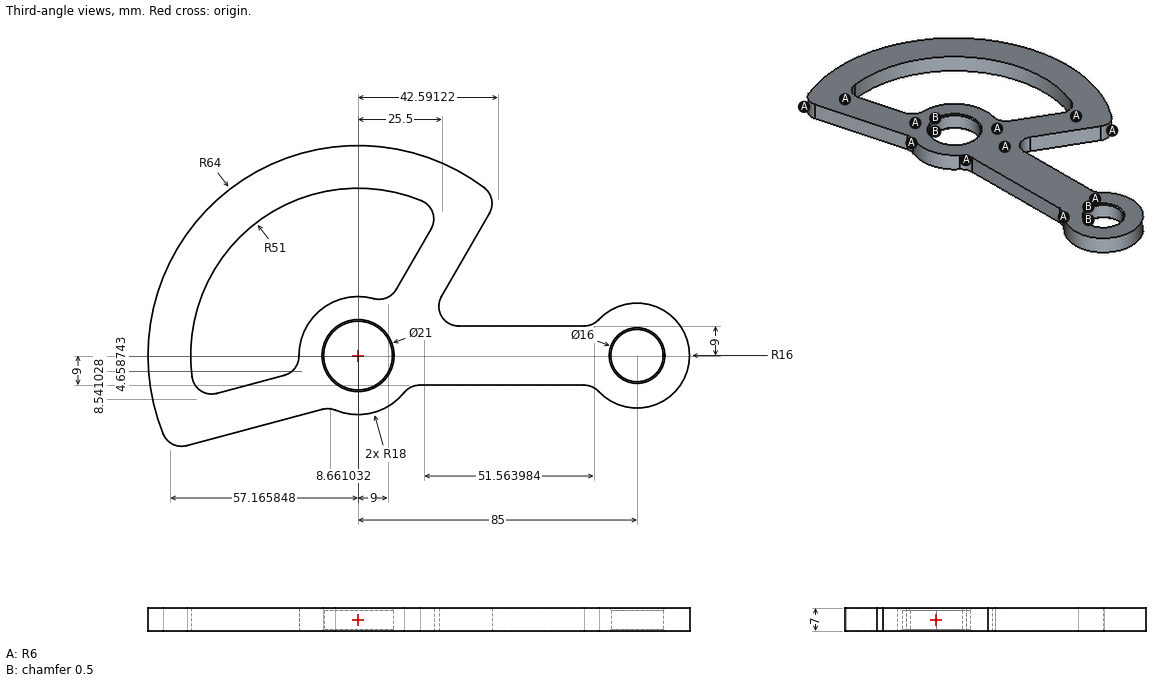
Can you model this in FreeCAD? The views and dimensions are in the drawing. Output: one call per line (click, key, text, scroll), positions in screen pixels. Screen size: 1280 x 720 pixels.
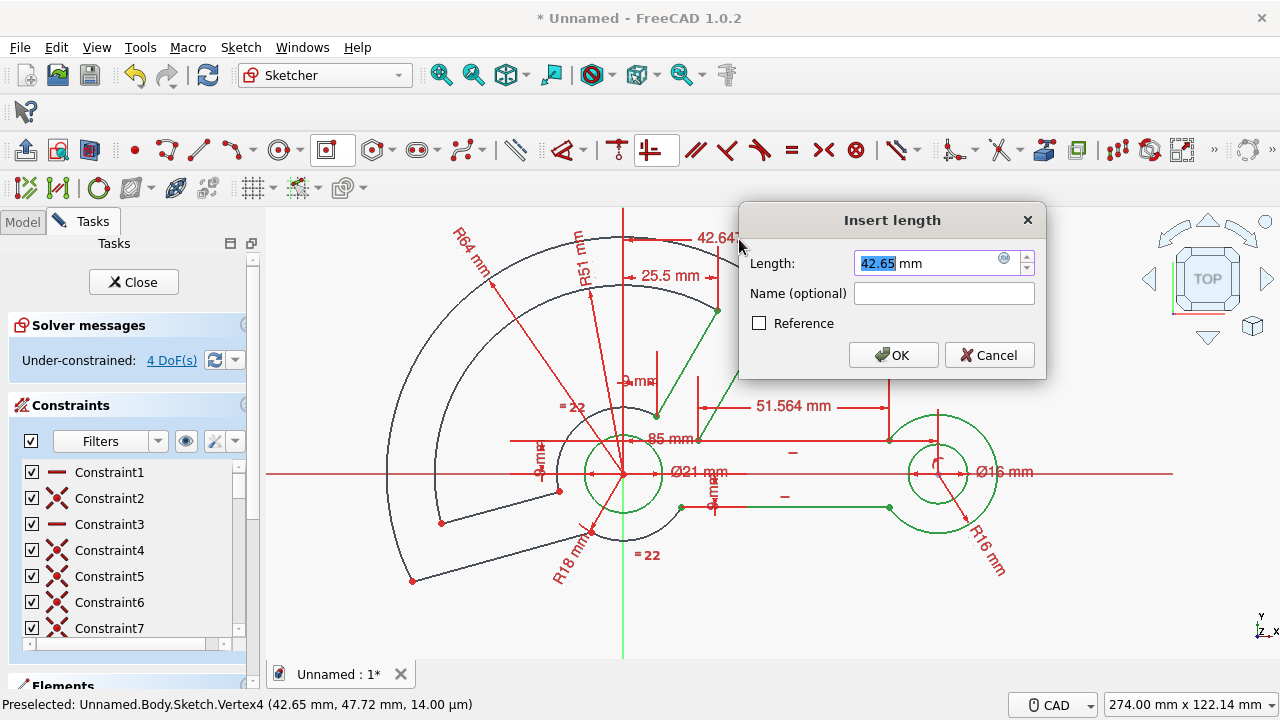
text(42.59122)
key(Return)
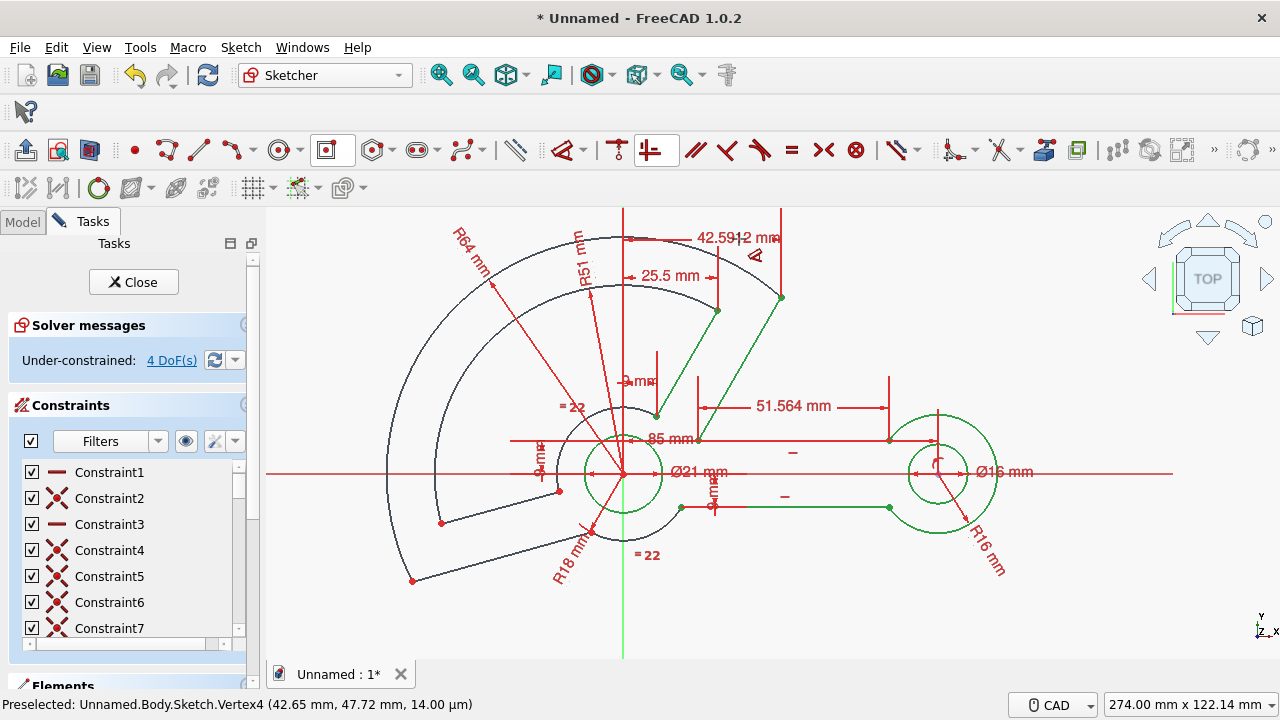
scroll(591, 532, up, 2)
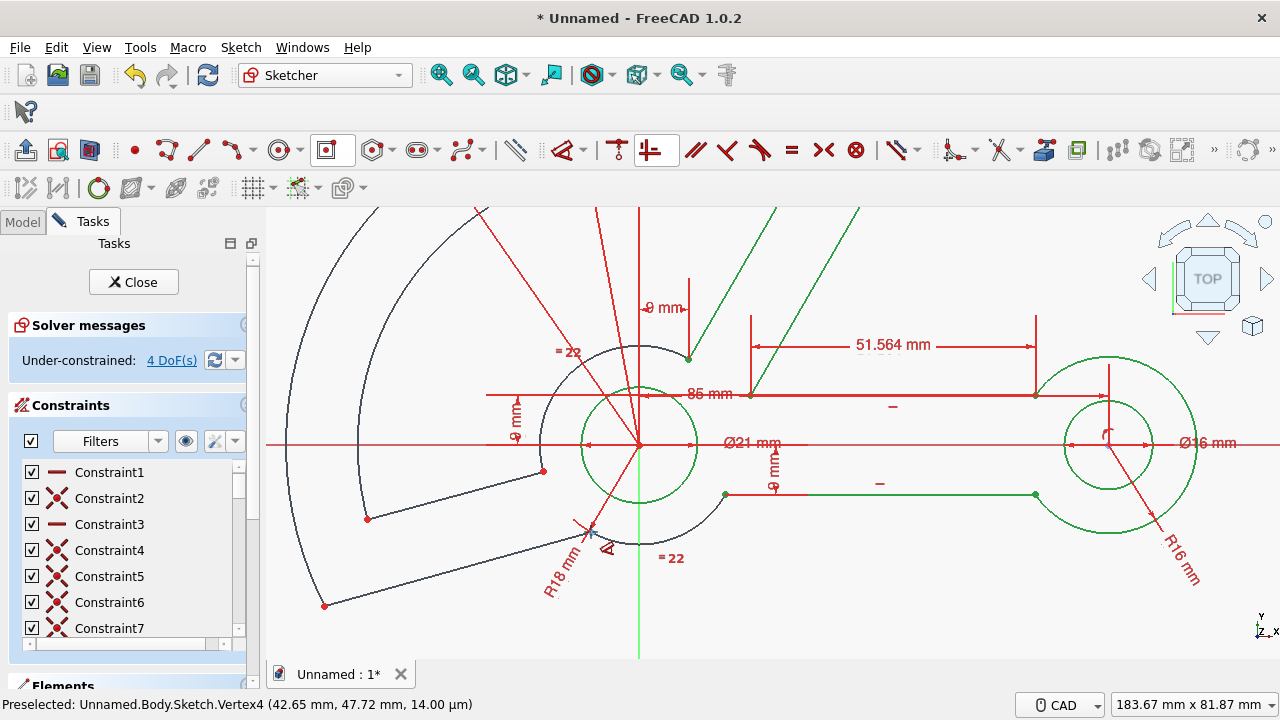
click(591, 532)
click(615, 411)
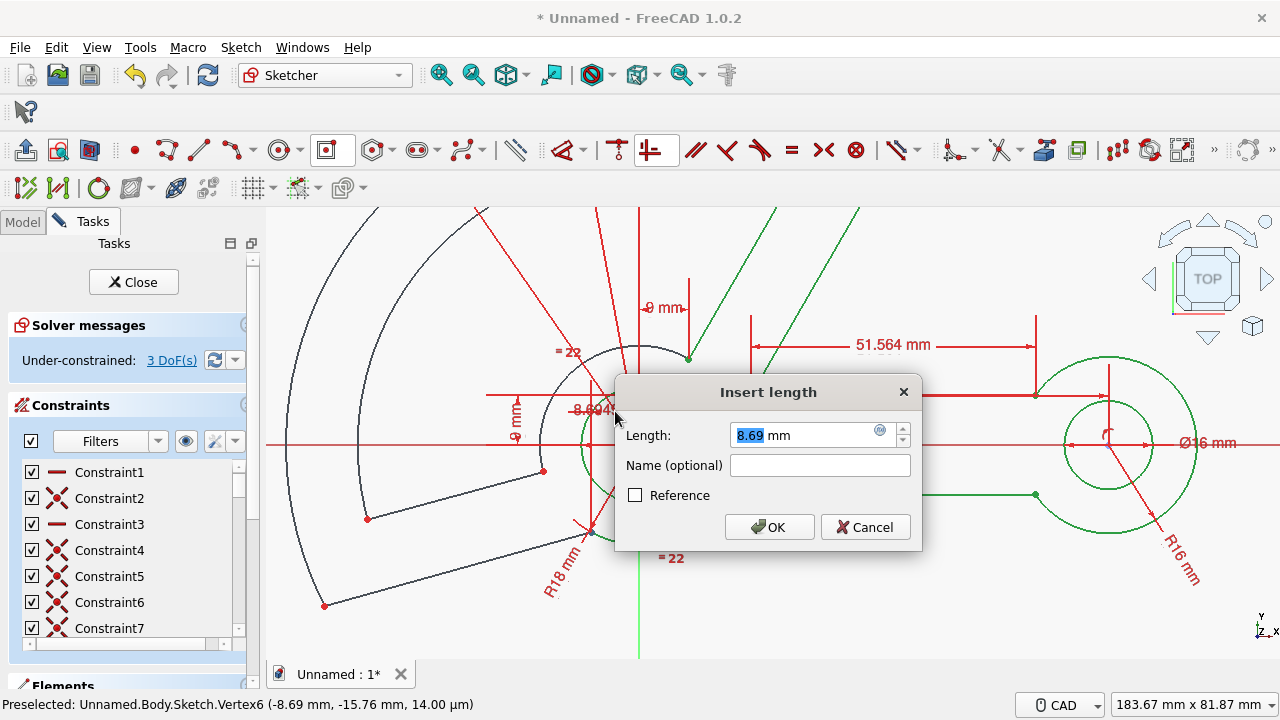
text(8.661032)
key(Return)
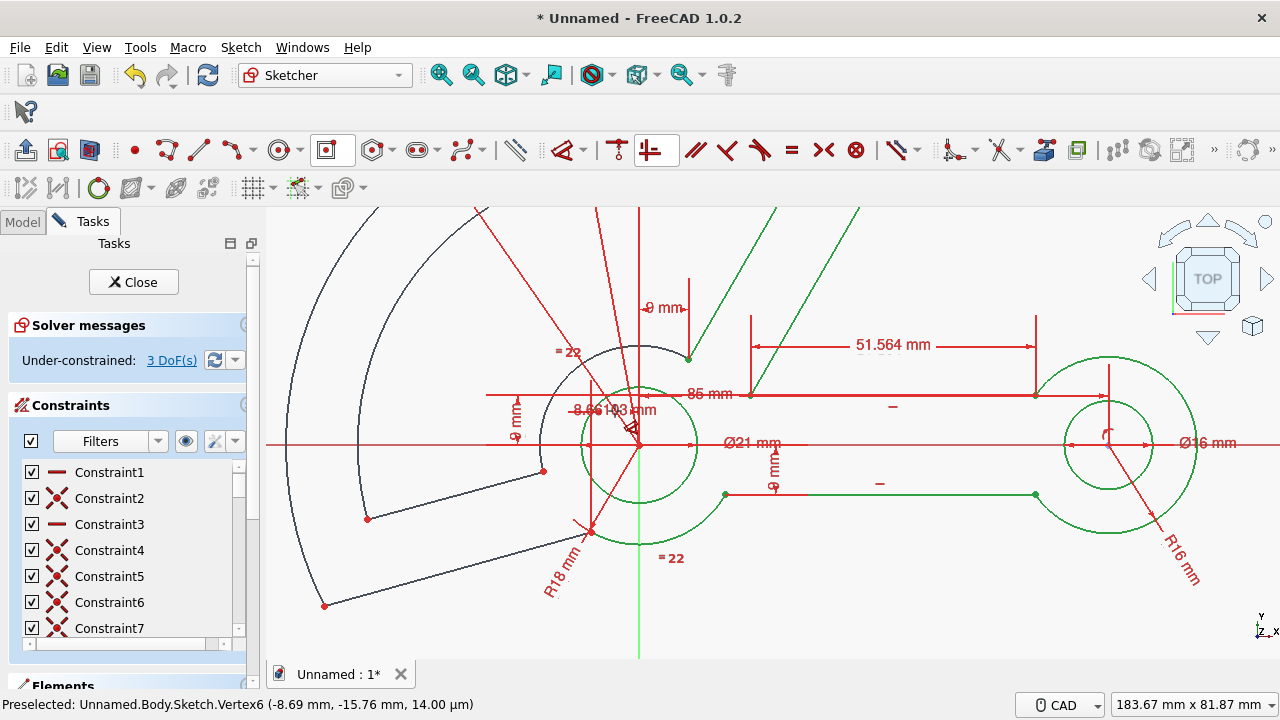
scroll(544, 472, up, 3)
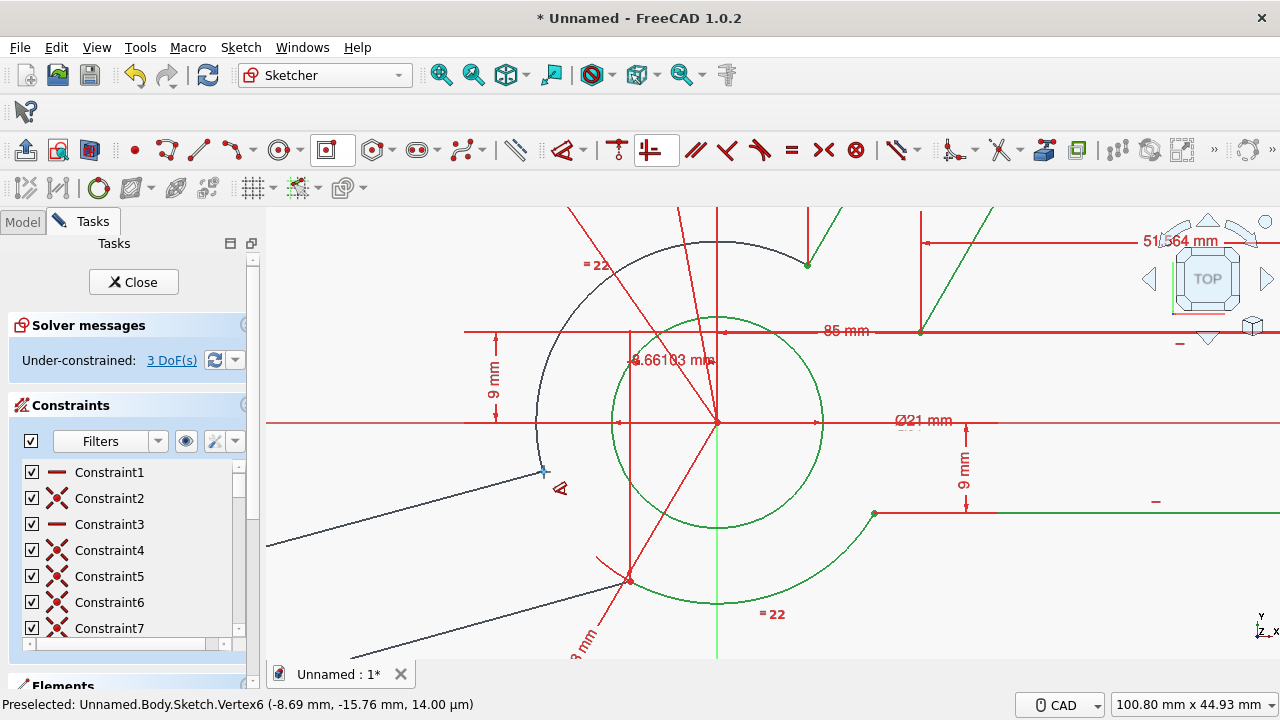
click(543, 471)
click(509, 447)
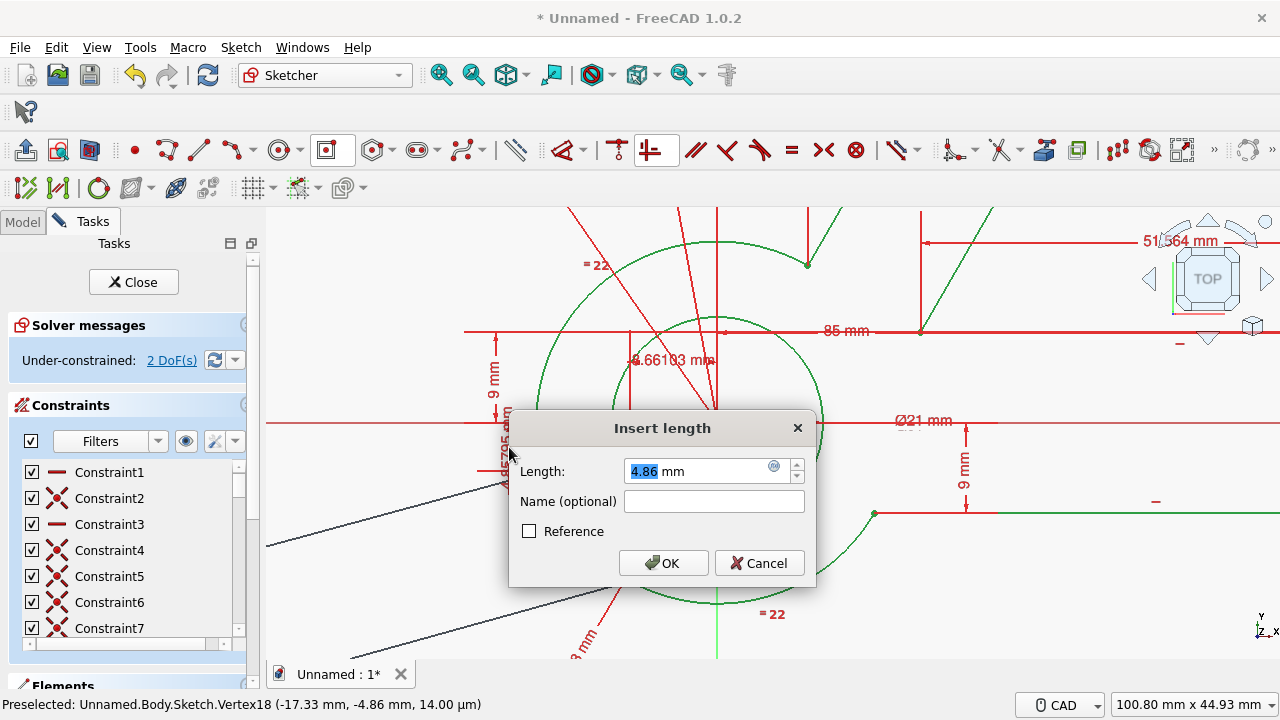
text(4.658743)
key(Return)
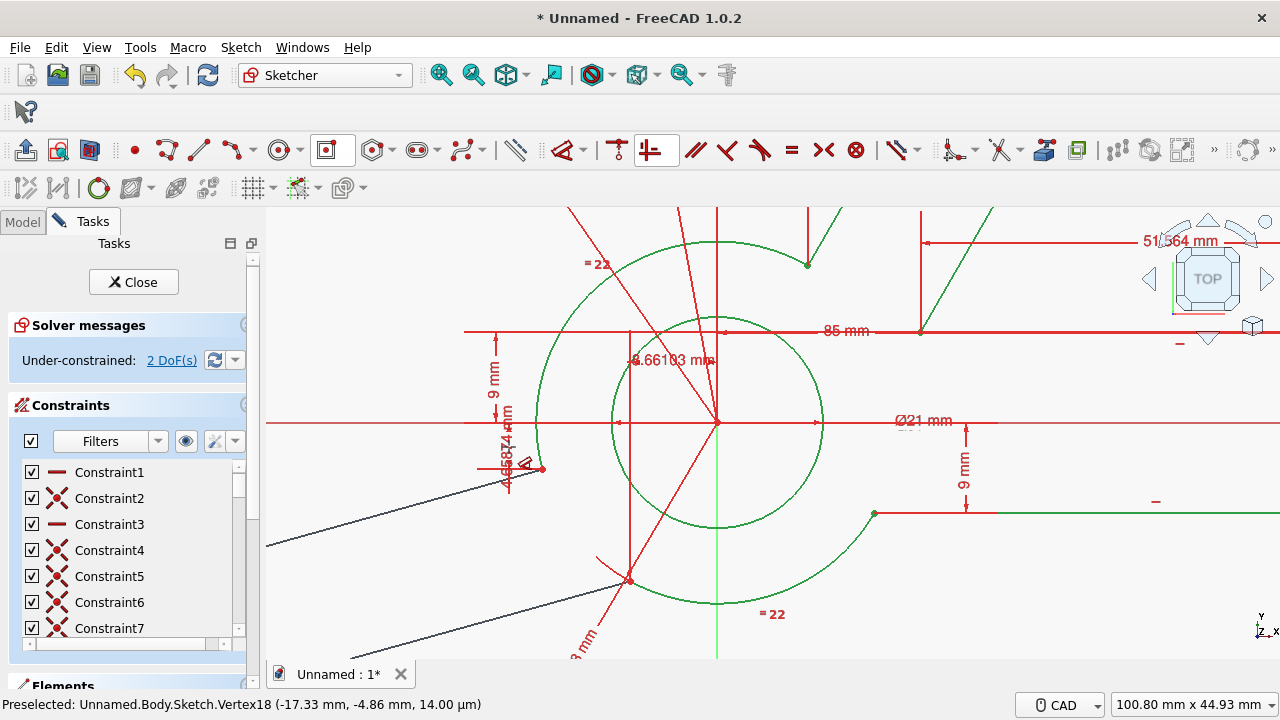
click(447, 496)
click(577, 514)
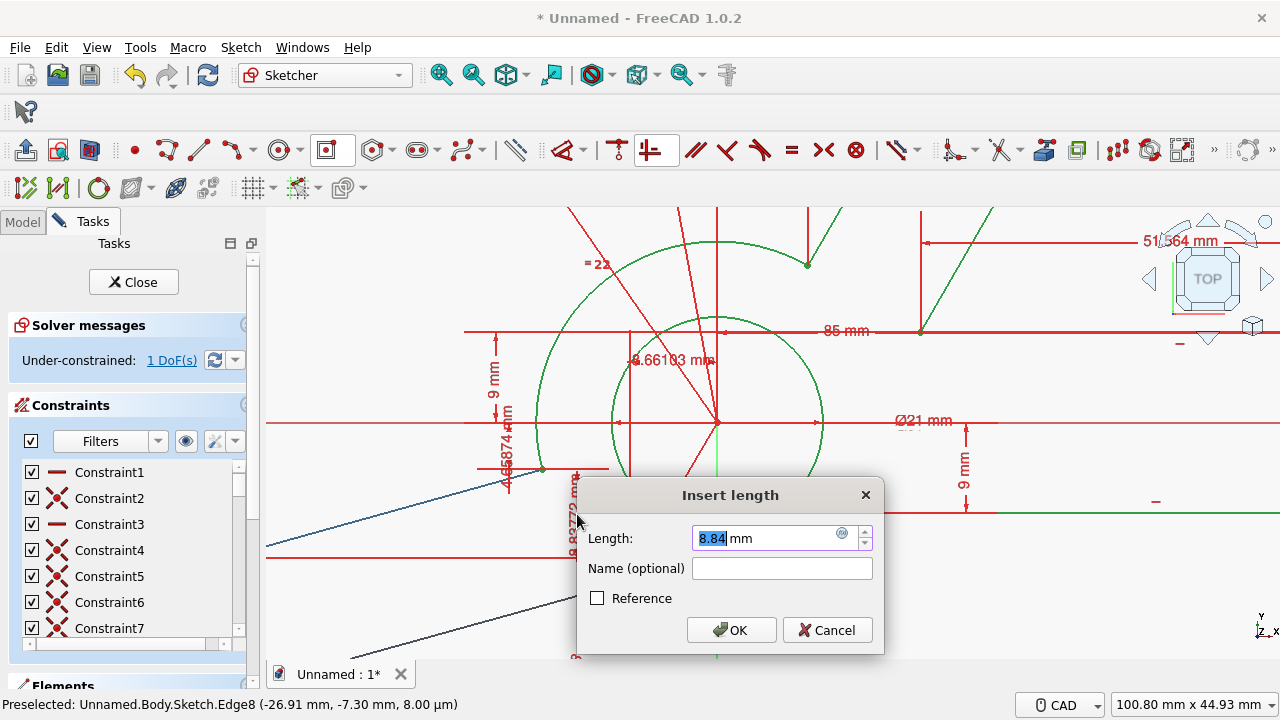
text(8.541028)
key(Return)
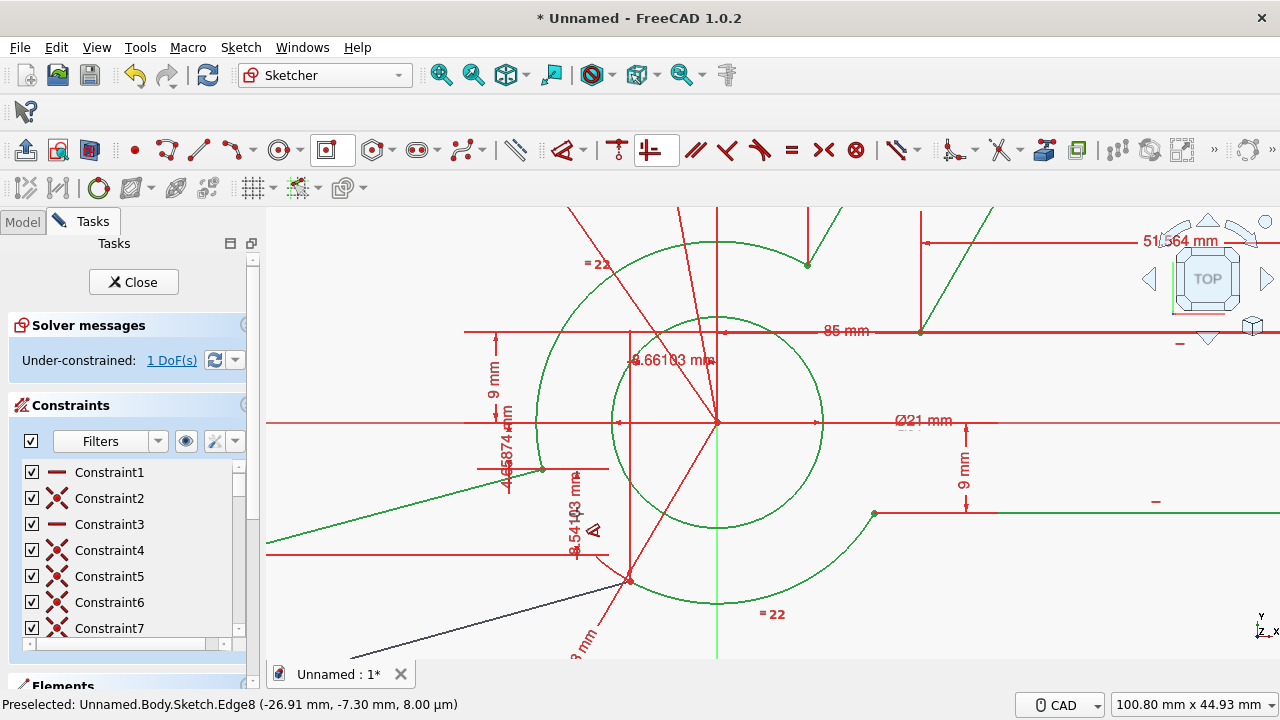
scroll(569, 503, down, 5)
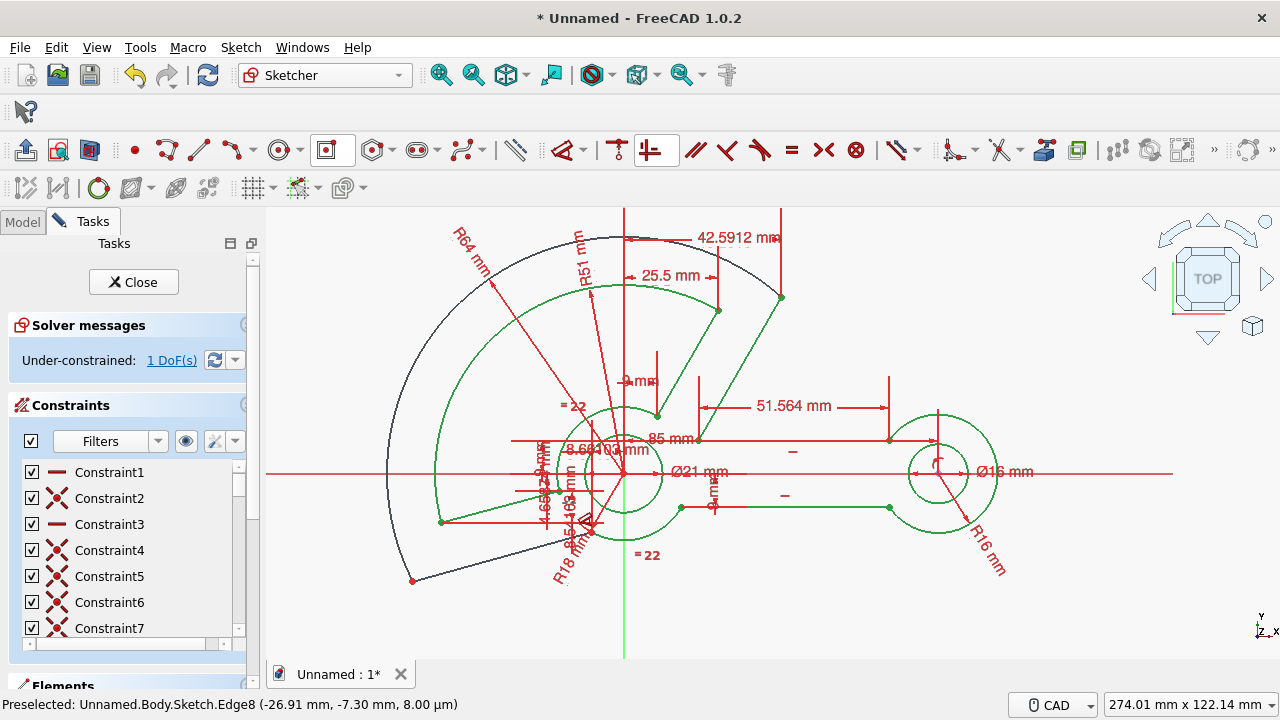
click(413, 582)
click(518, 616)